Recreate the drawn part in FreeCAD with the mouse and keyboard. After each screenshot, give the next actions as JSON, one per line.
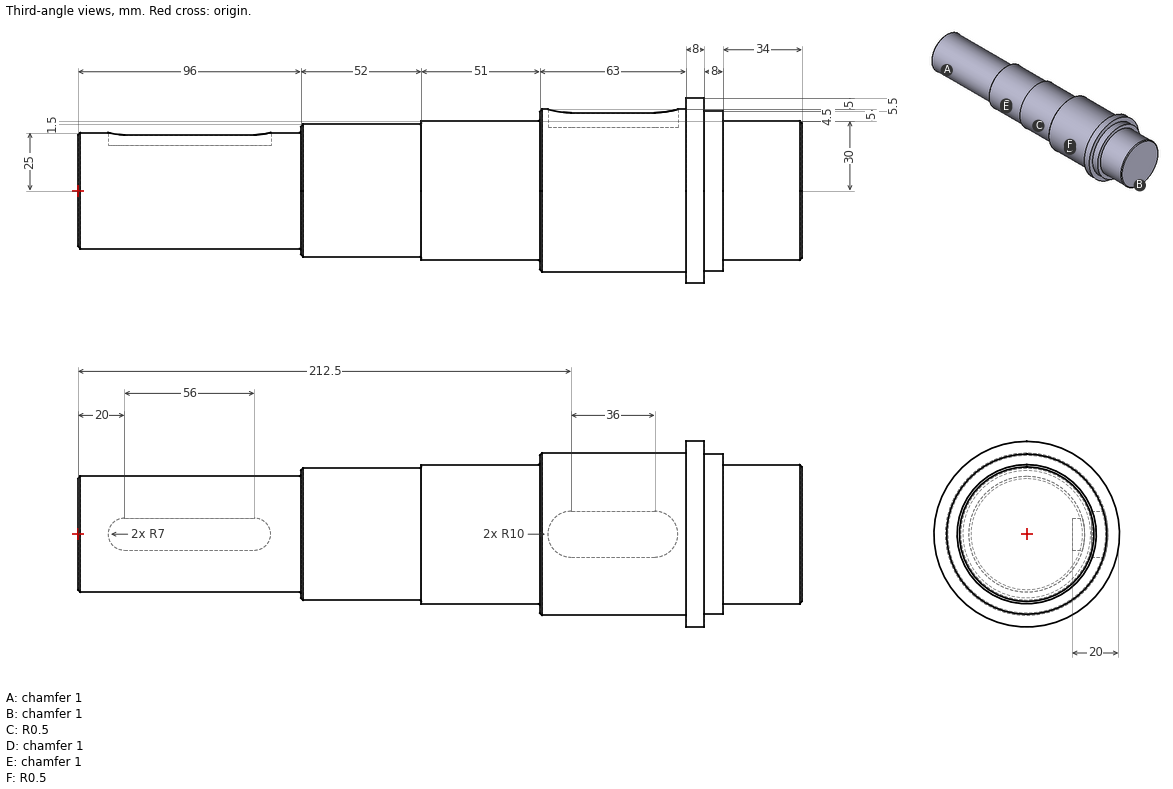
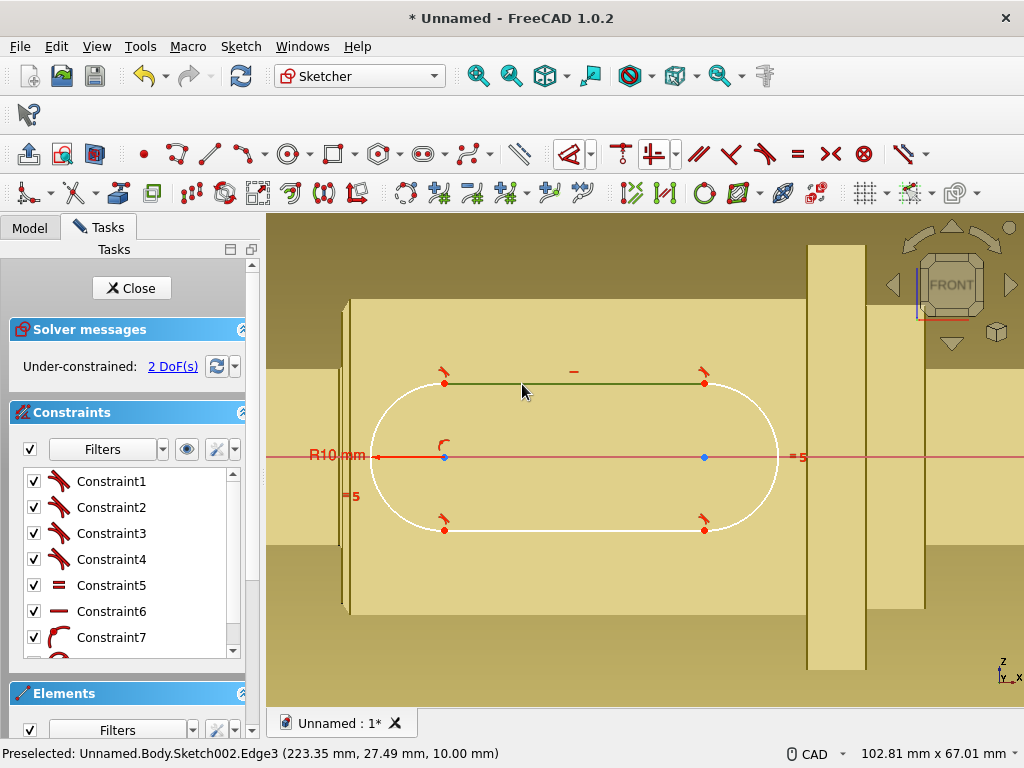
{"action": "left_click", "coordinate": [590, 154]}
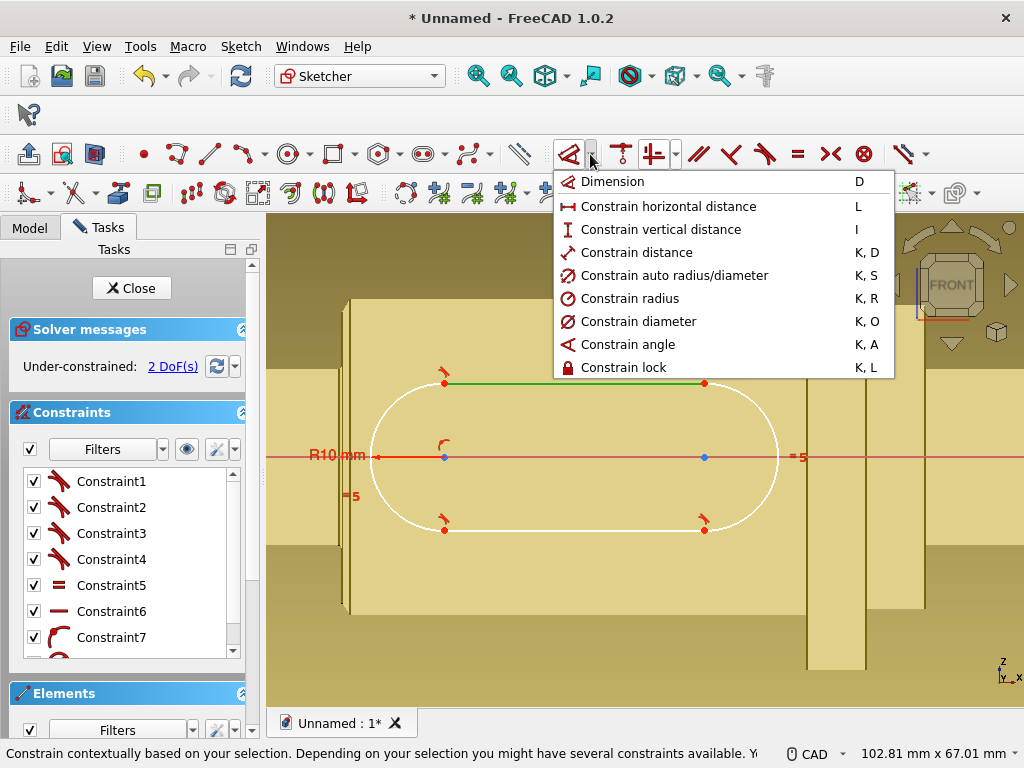
{"action": "left_click", "coordinate": [724, 206]}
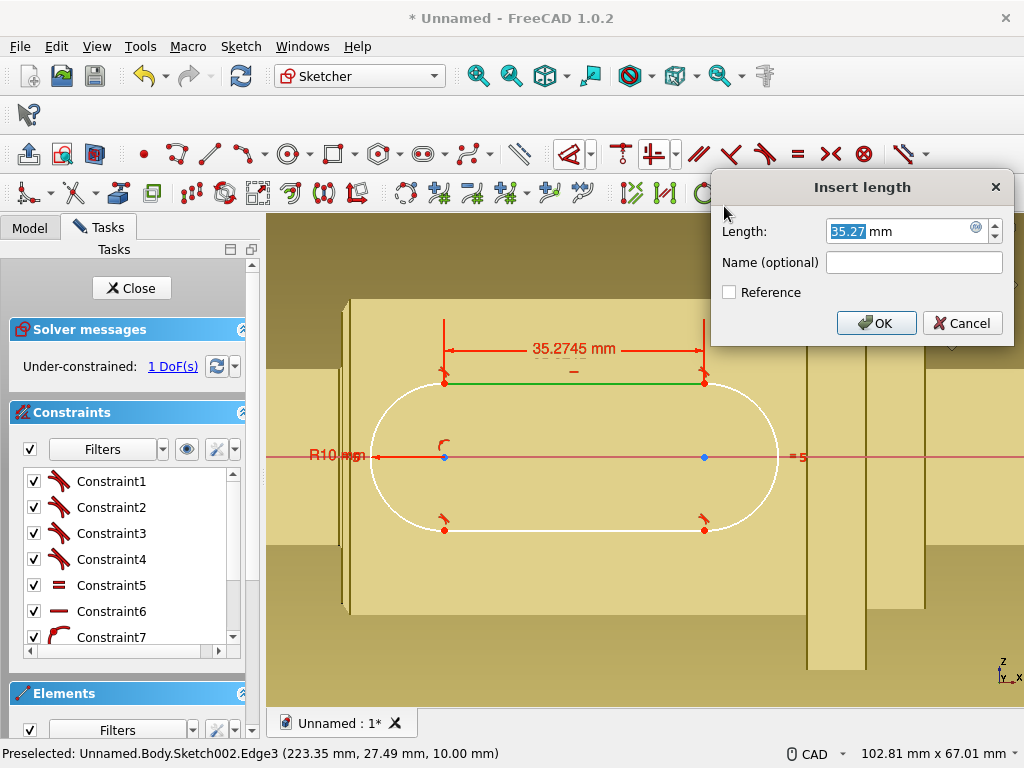
{"action": "type", "text": "36"}
{"action": "key", "text": "Return"}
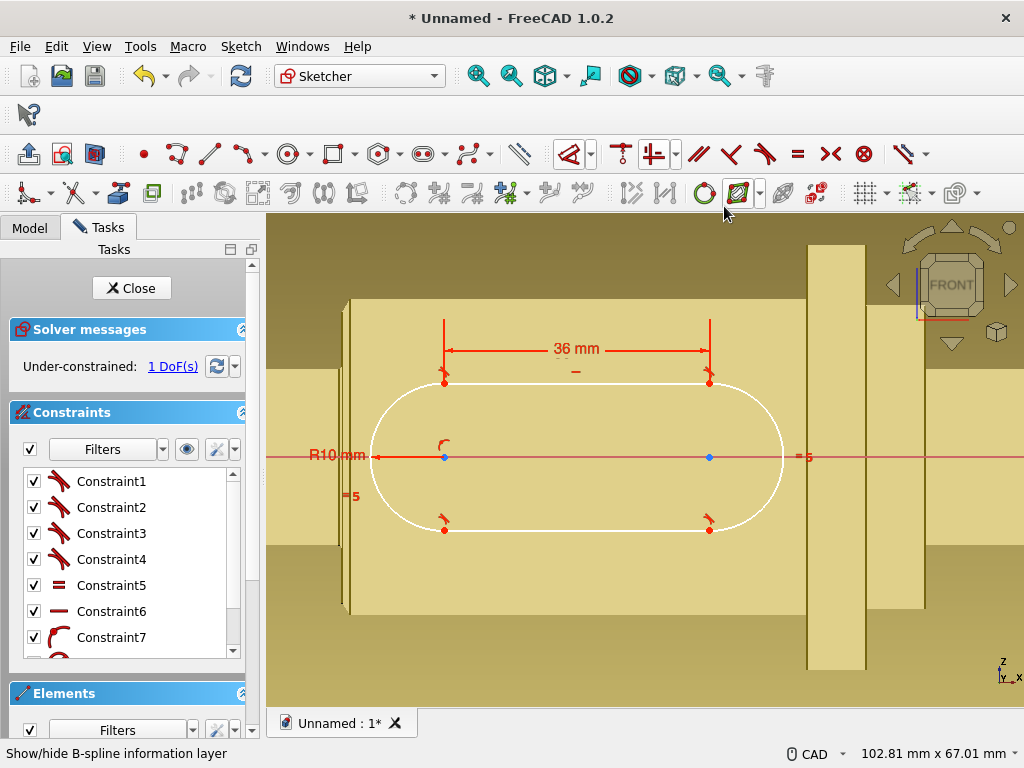
{"action": "left_click", "coordinate": [444, 384]}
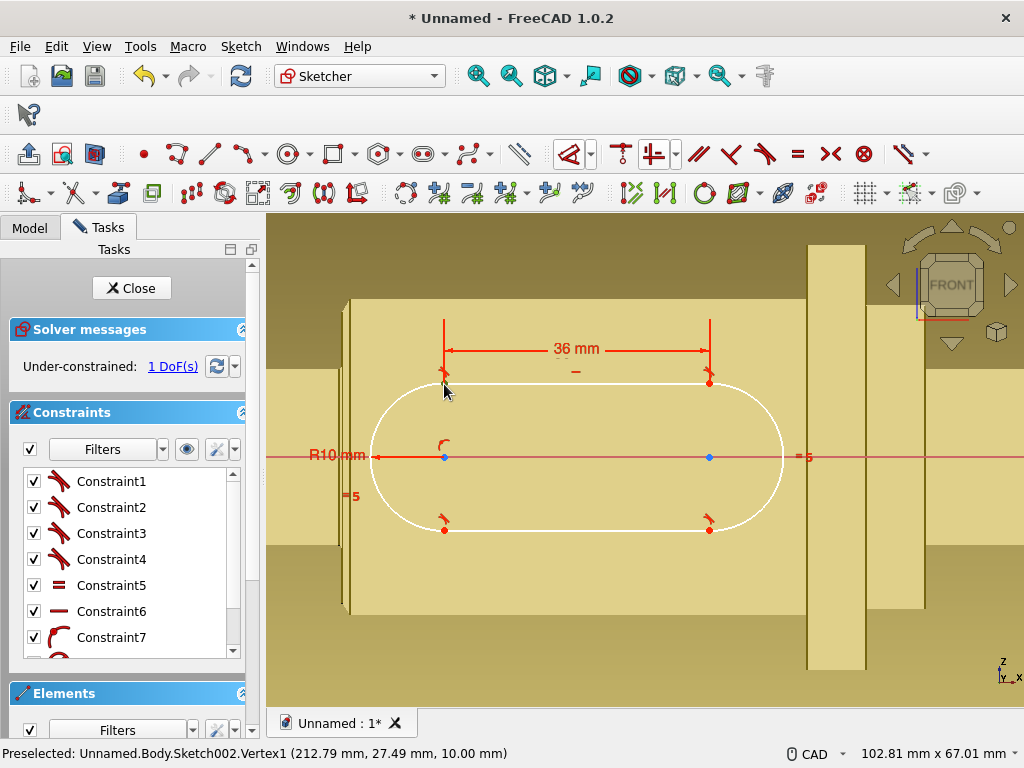
{"action": "key", "text": "l"}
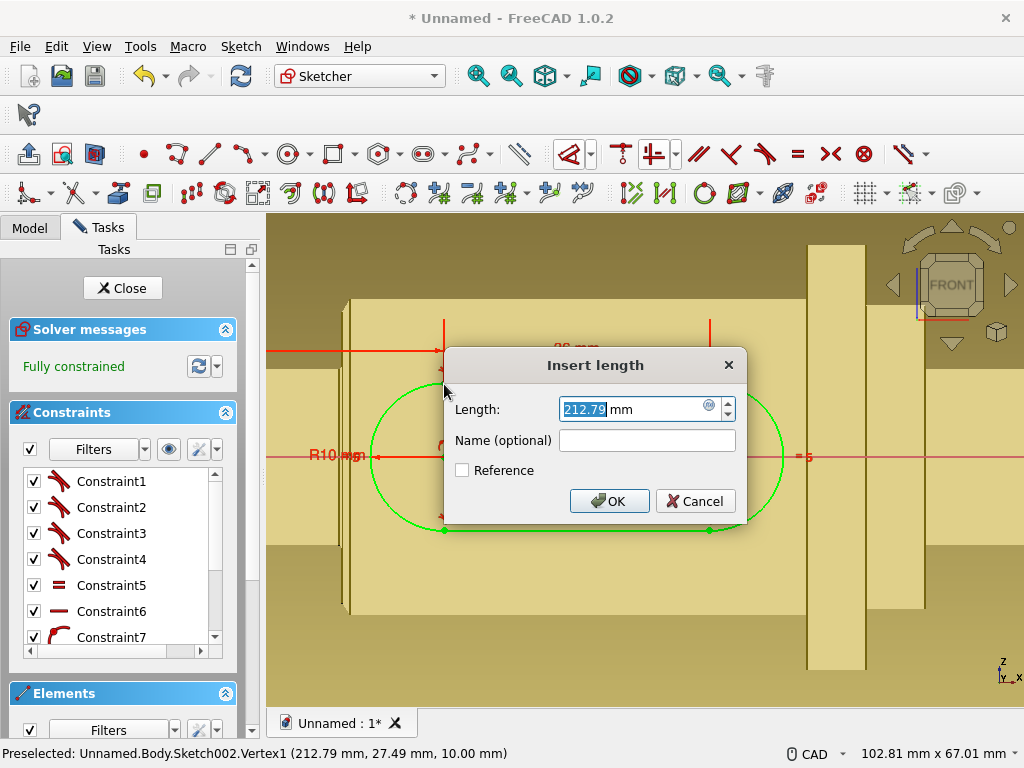
{"action": "type", "text": "212.5"}
{"action": "key", "text": "Return"}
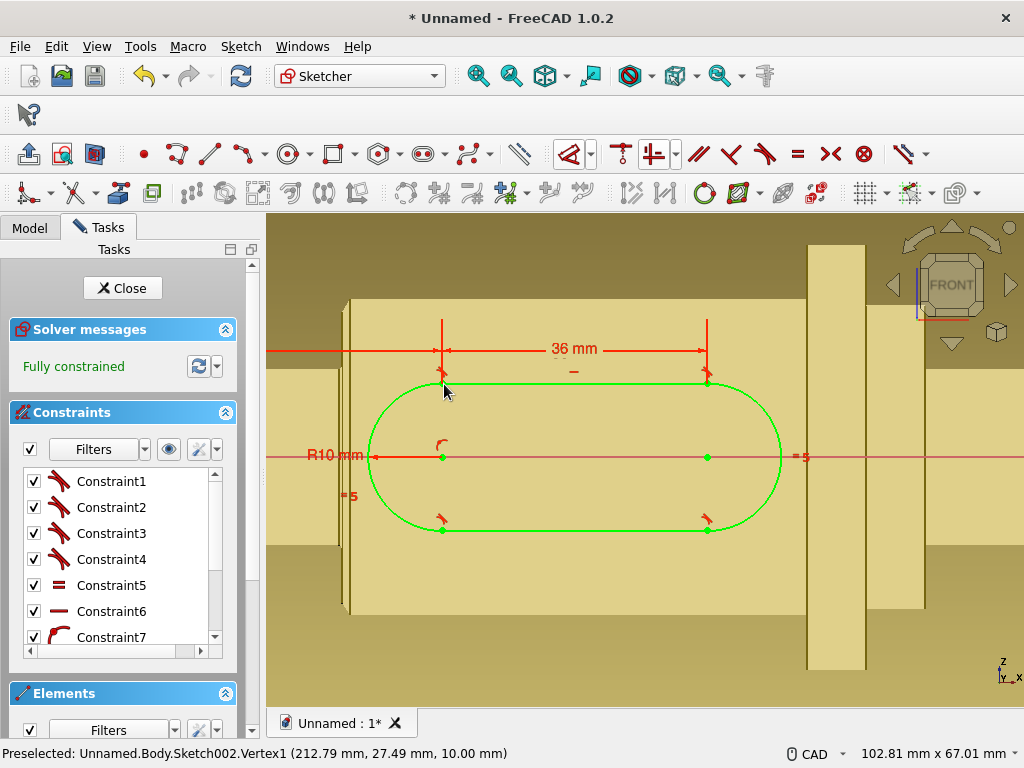
{"action": "left_click", "coordinate": [123, 288]}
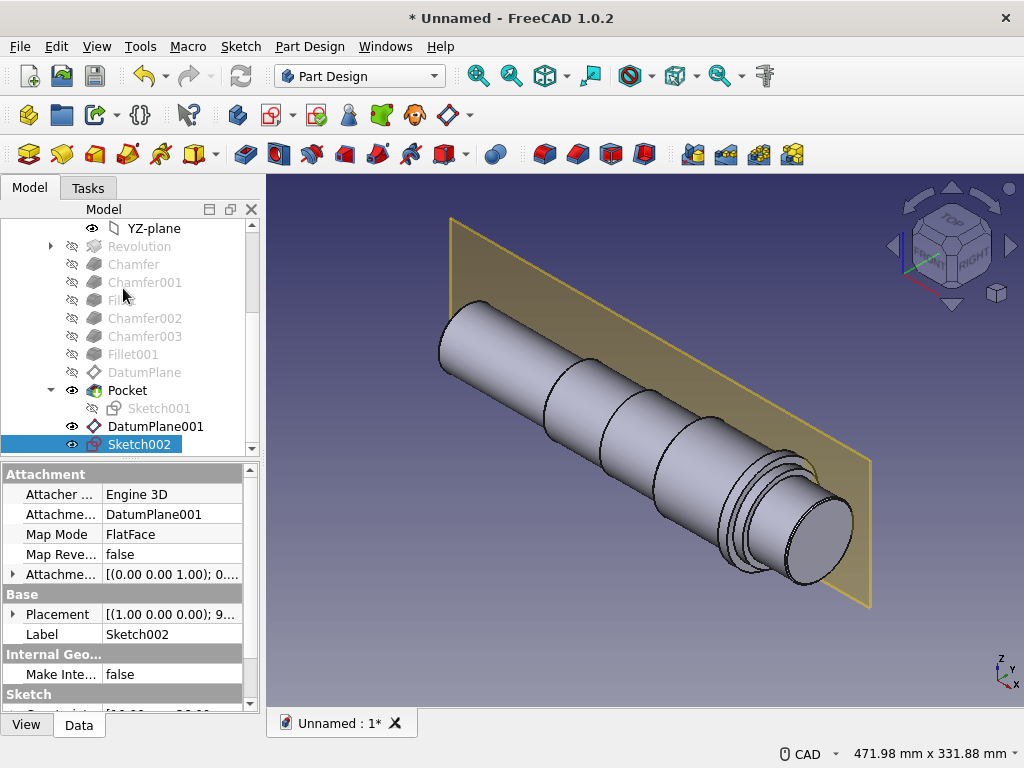
{"action": "left_click", "coordinate": [246, 154]}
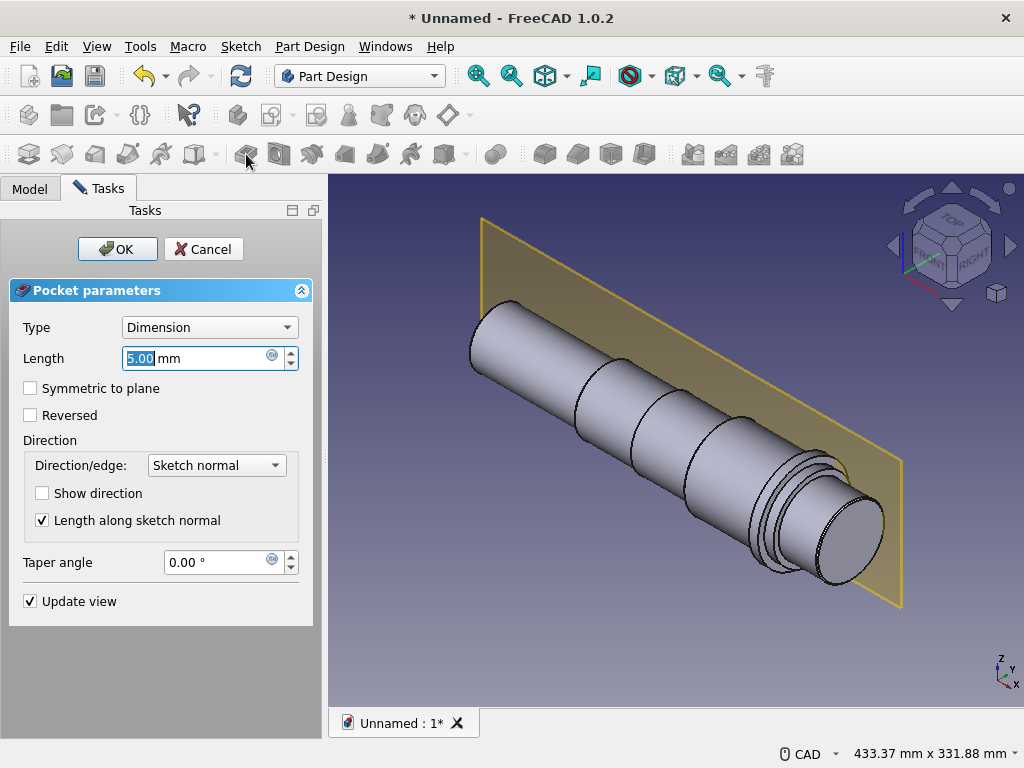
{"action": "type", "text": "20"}
{"action": "key", "text": "Tab"}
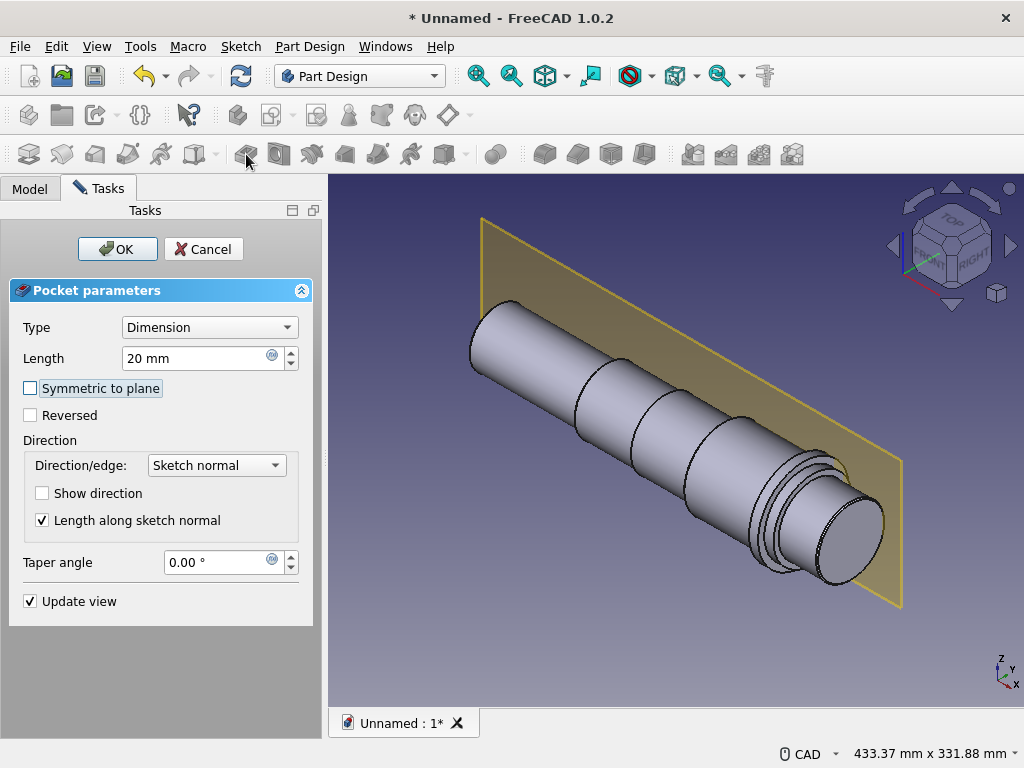
{"action": "left_click", "coordinate": [118, 249]}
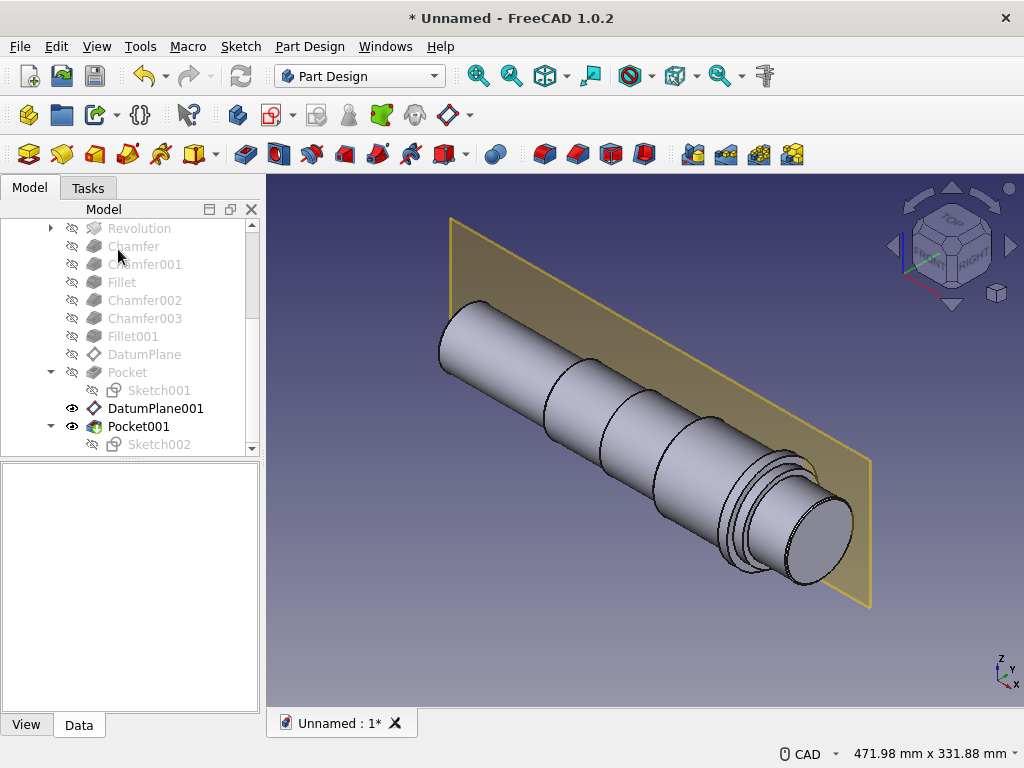
{"action": "left_click", "coordinate": [117, 408]}
{"action": "key", "text": "space"}